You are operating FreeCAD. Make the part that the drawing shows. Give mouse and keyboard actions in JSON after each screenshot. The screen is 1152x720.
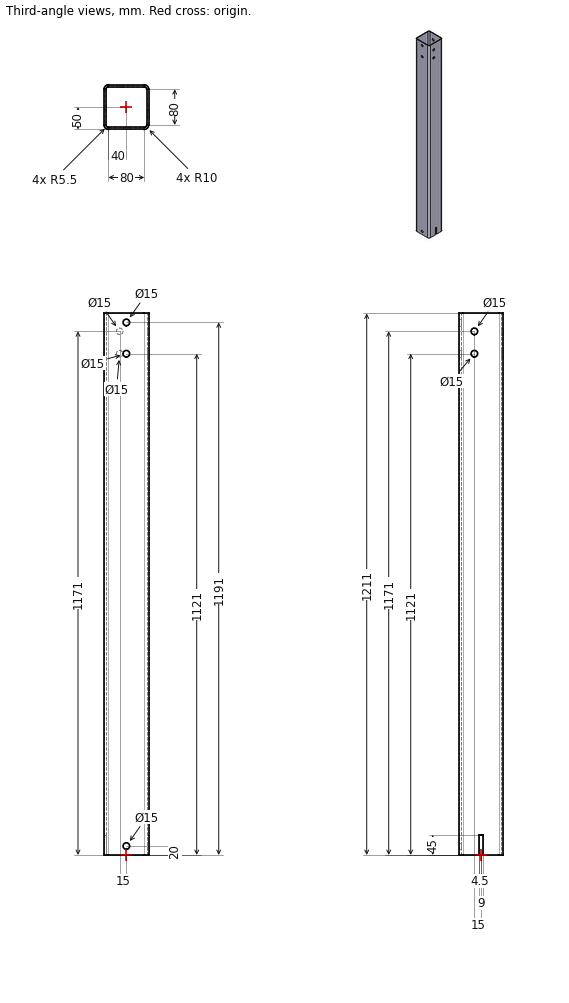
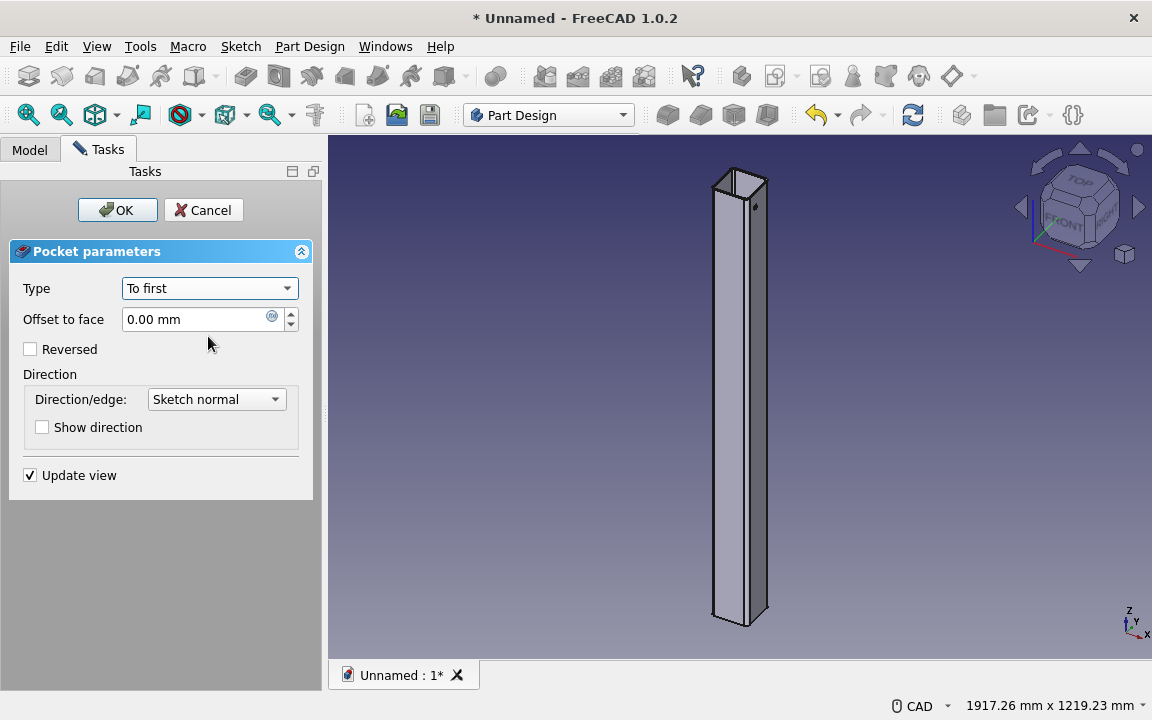
{"action": "left_click", "coordinate": [118, 210]}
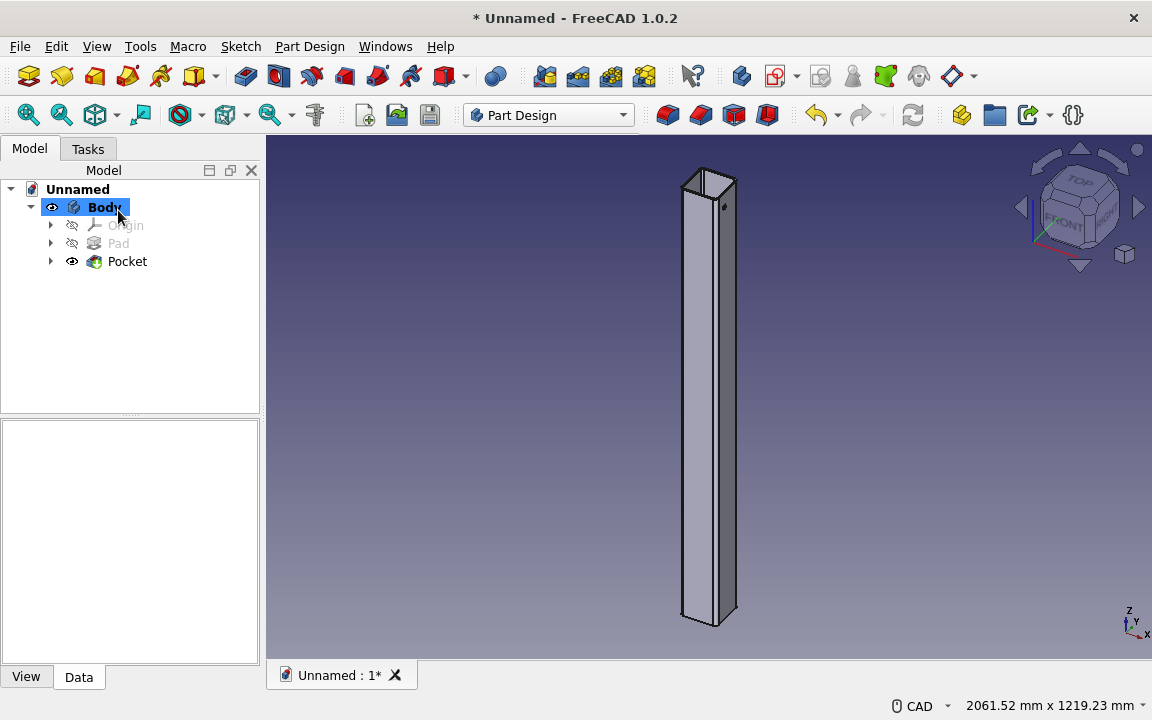
{"action": "left_click", "coordinate": [728, 219]}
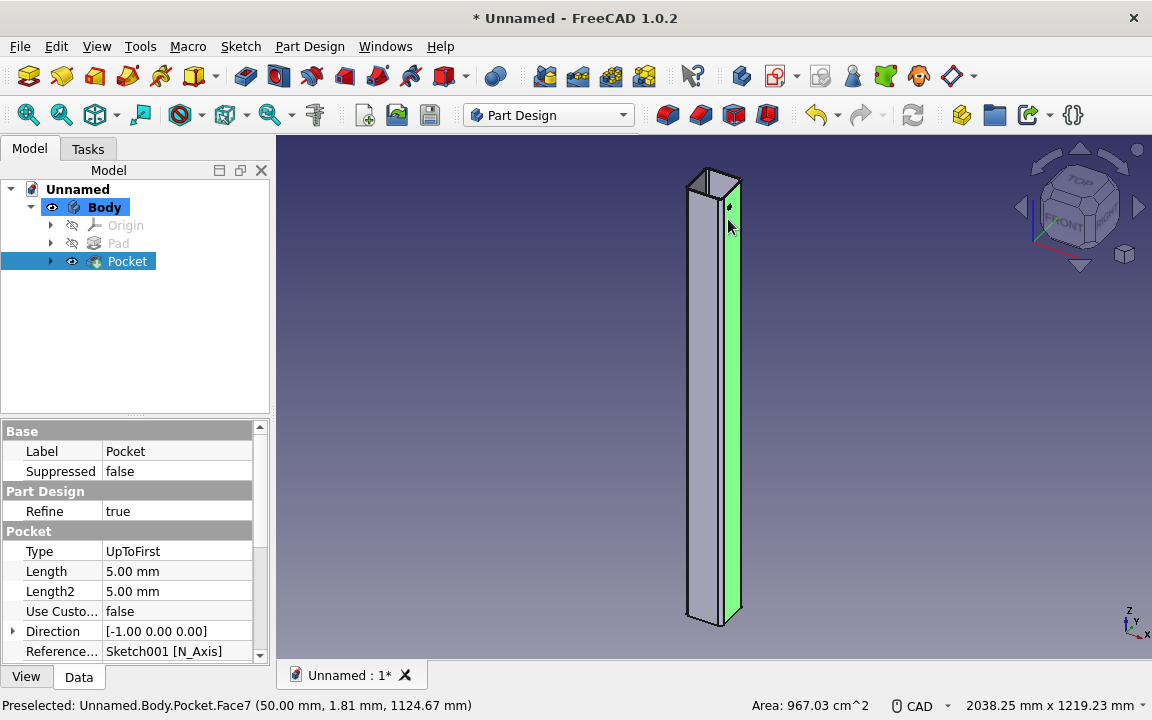
{"action": "left_click", "coordinate": [774, 76]}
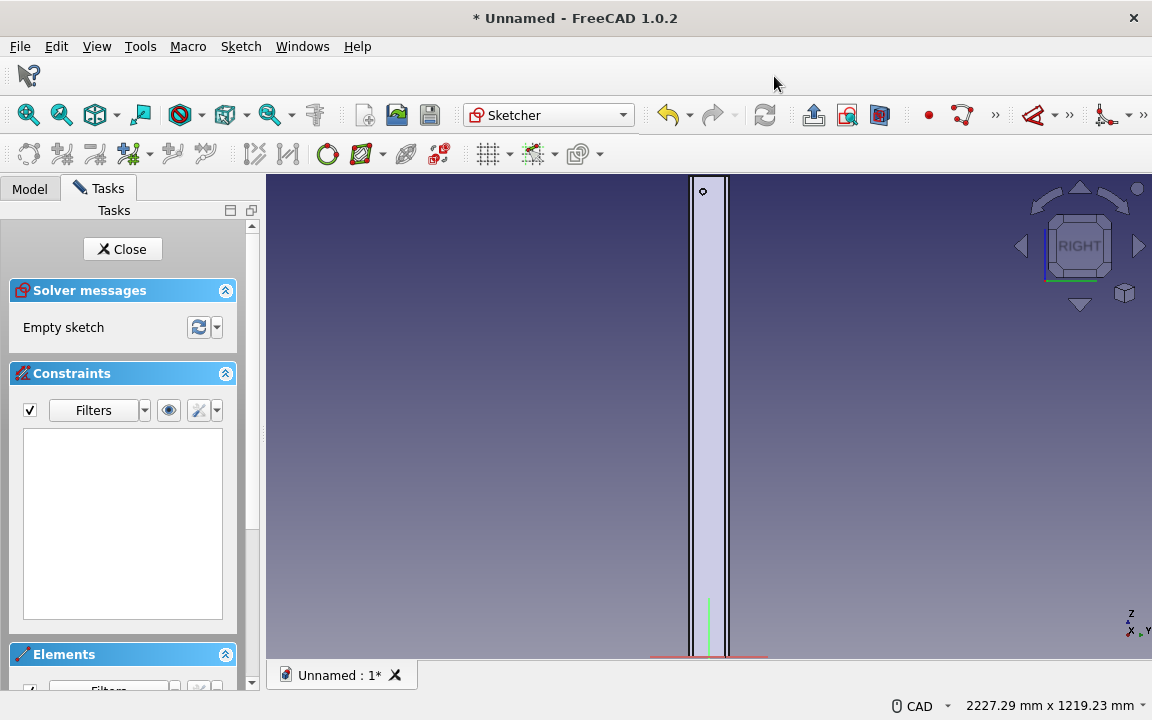
{"action": "scroll", "coordinate": [706, 202], "scroll_direction": "up", "scroll_amount": 15}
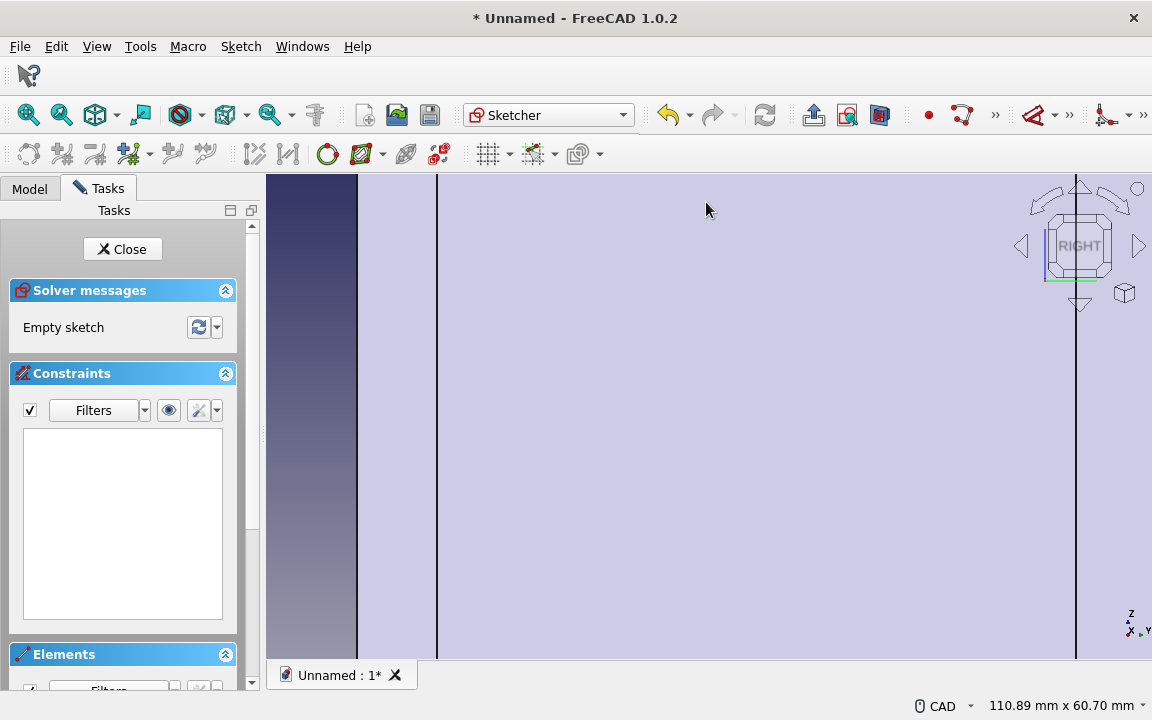
{"action": "scroll", "coordinate": [635, 375], "scroll_direction": "up", "scroll_amount": 5}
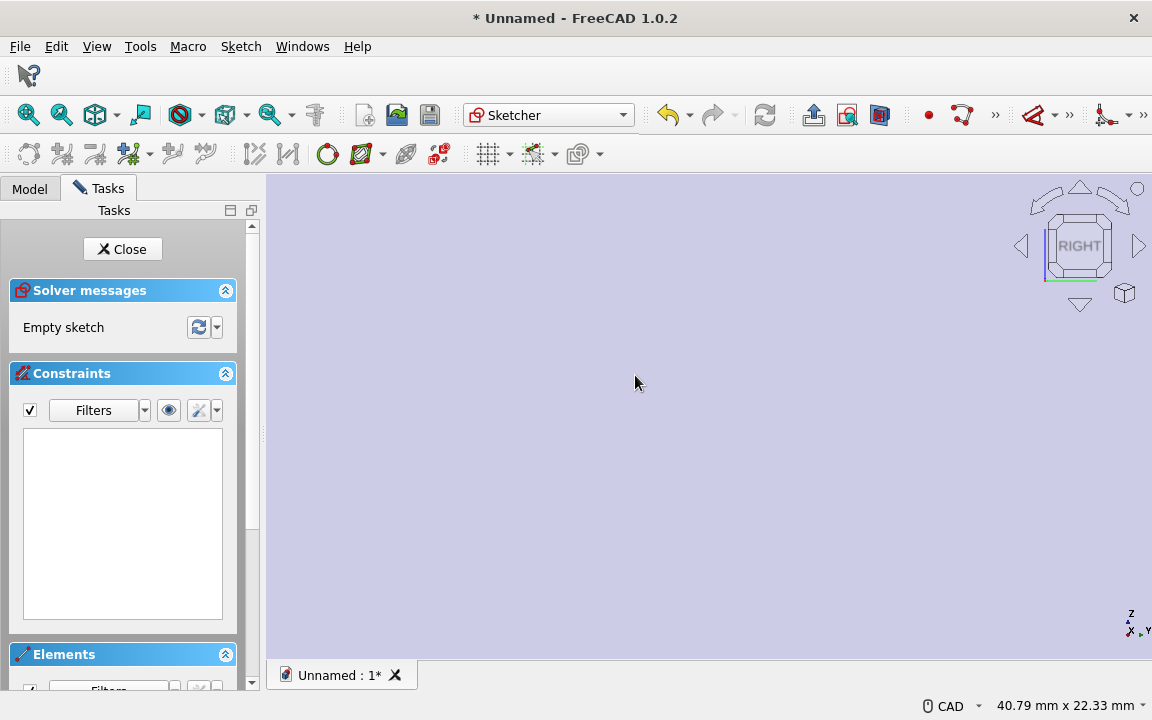
{"action": "key", "text": "g c"}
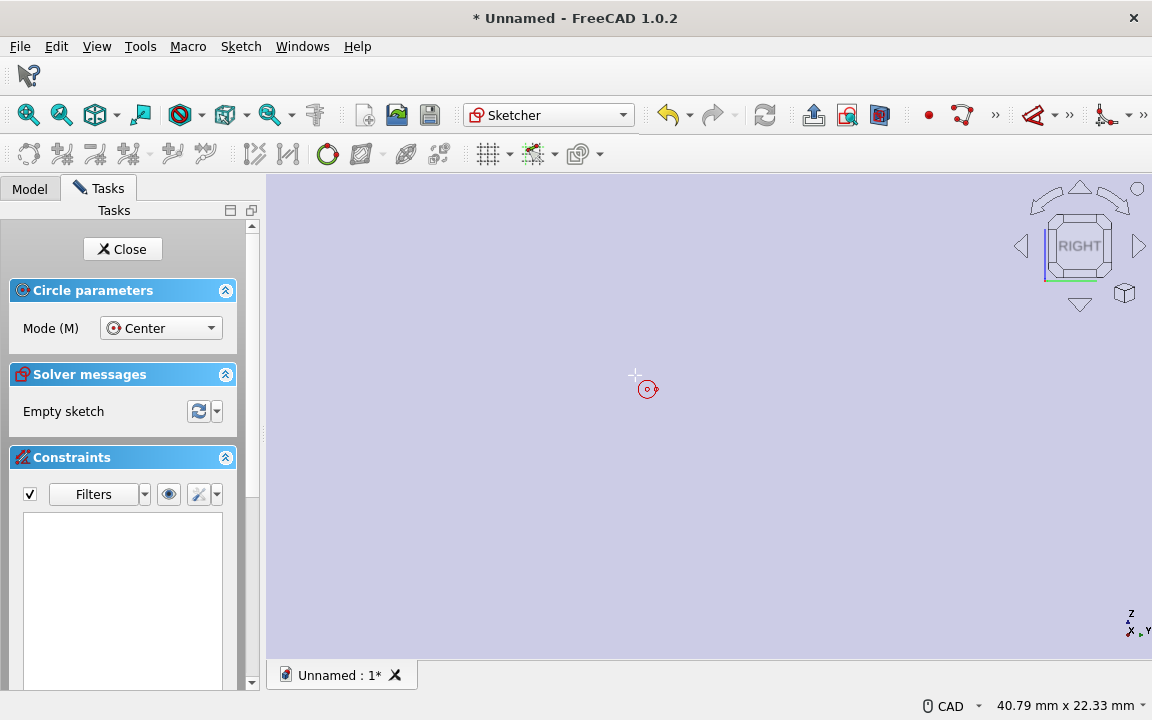
{"action": "left_click", "coordinate": [640, 416]}
{"action": "left_click", "coordinate": [755, 301]}
{"action": "key", "text": "Escape"}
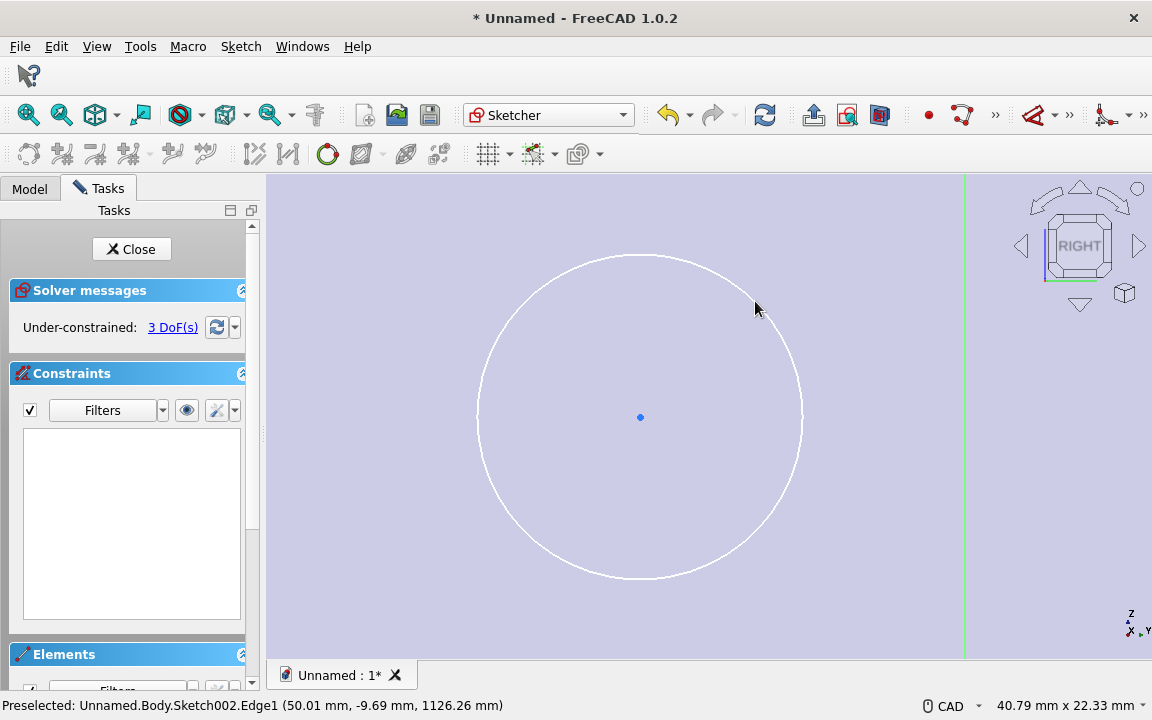
{"action": "key", "text": "d"}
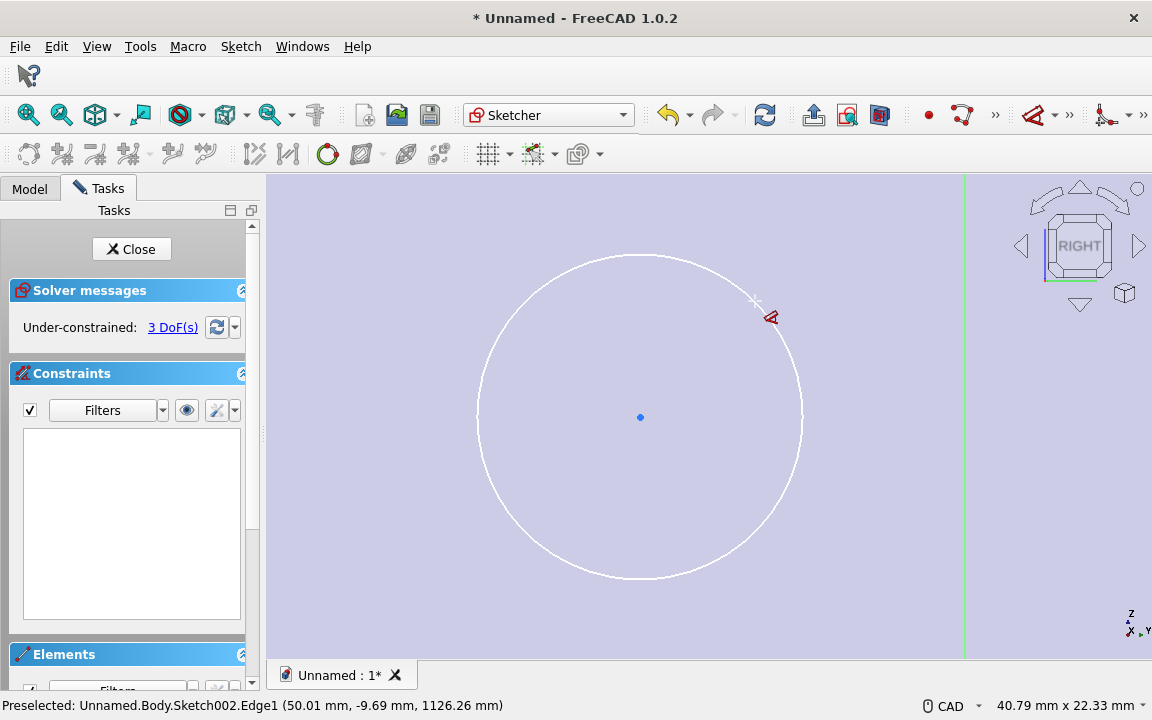
{"action": "left_click", "coordinate": [755, 302]}
{"action": "left_click", "coordinate": [778, 279]}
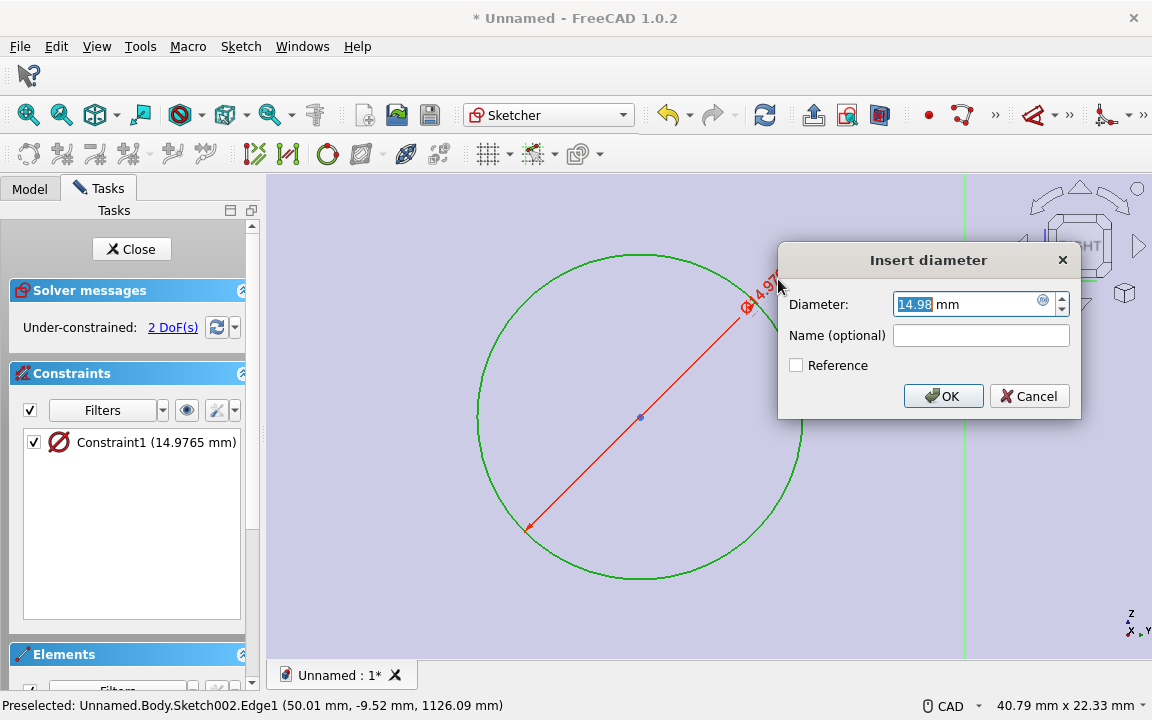
{"action": "type", "text": "15"}
{"action": "key", "text": "Return"}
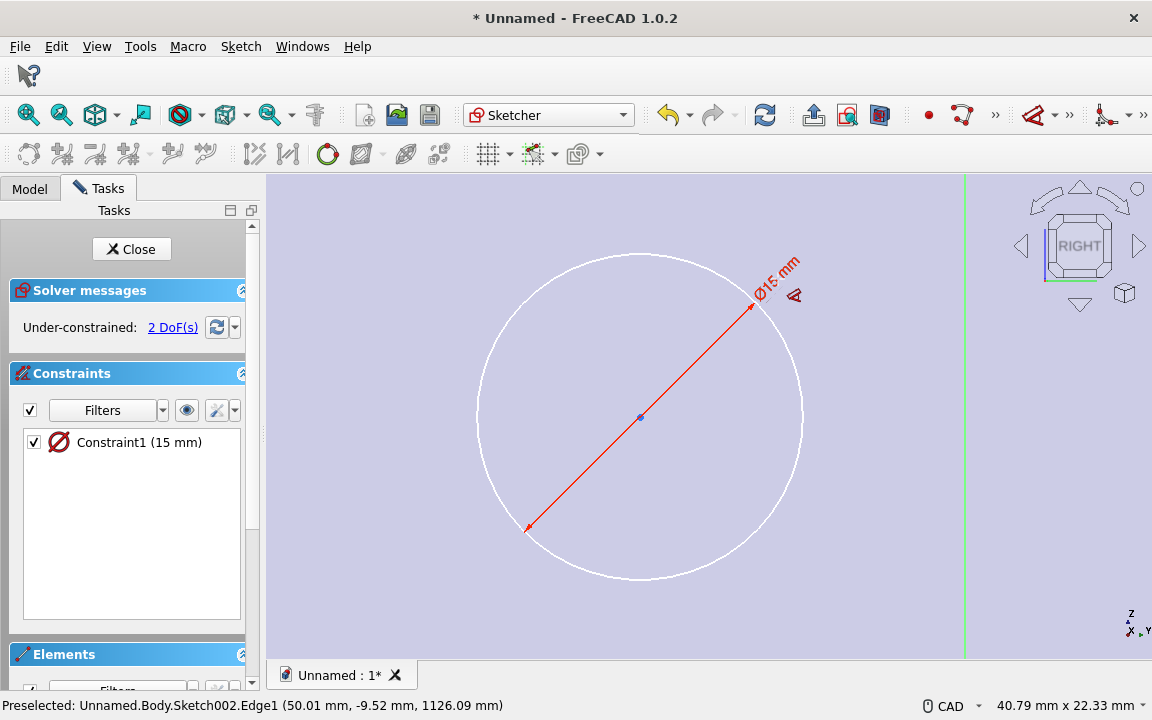
{"action": "left_click", "coordinate": [640, 417]}
{"action": "left_click", "coordinate": [728, 383]}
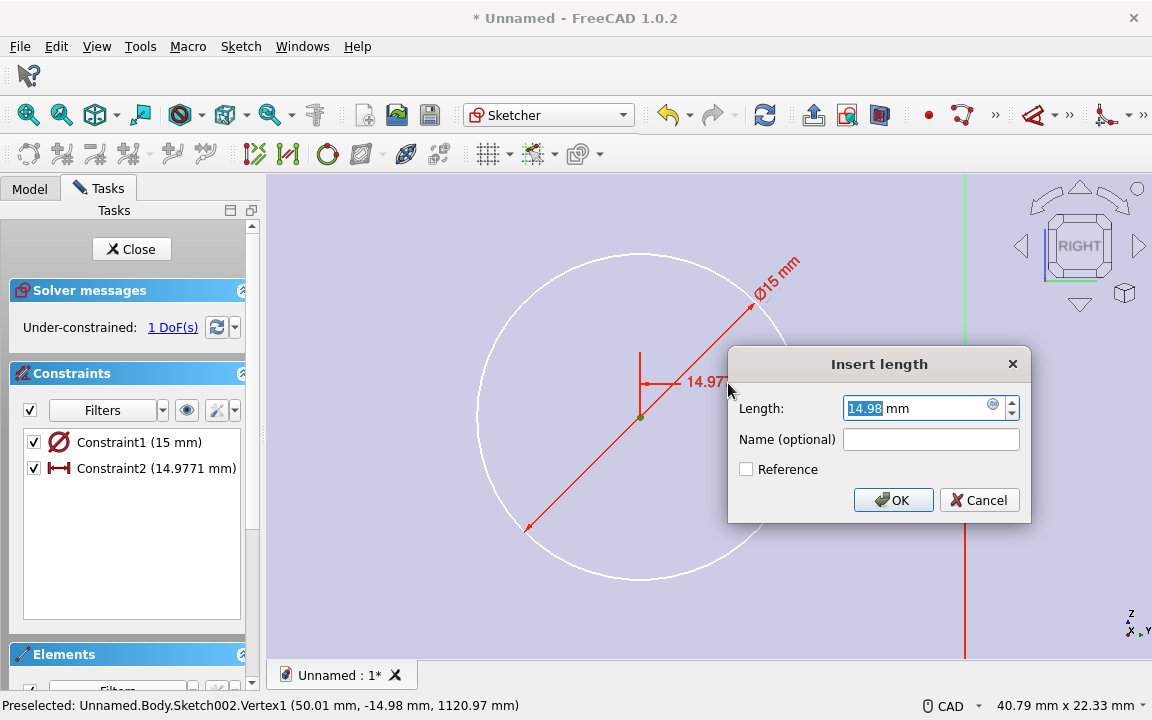
{"action": "type", "text": "15"}
{"action": "key", "text": "Return"}